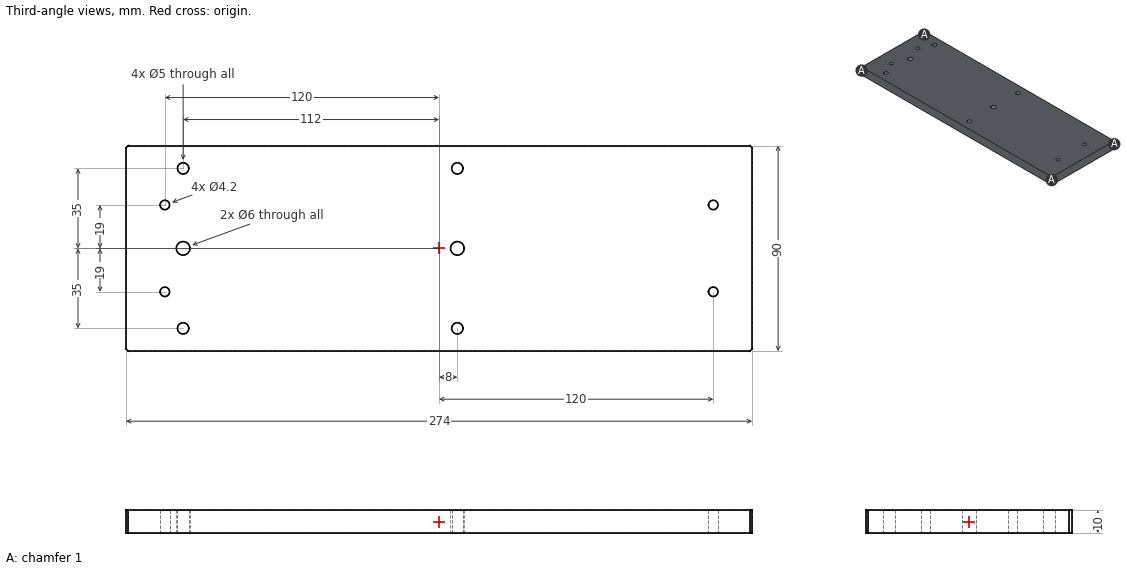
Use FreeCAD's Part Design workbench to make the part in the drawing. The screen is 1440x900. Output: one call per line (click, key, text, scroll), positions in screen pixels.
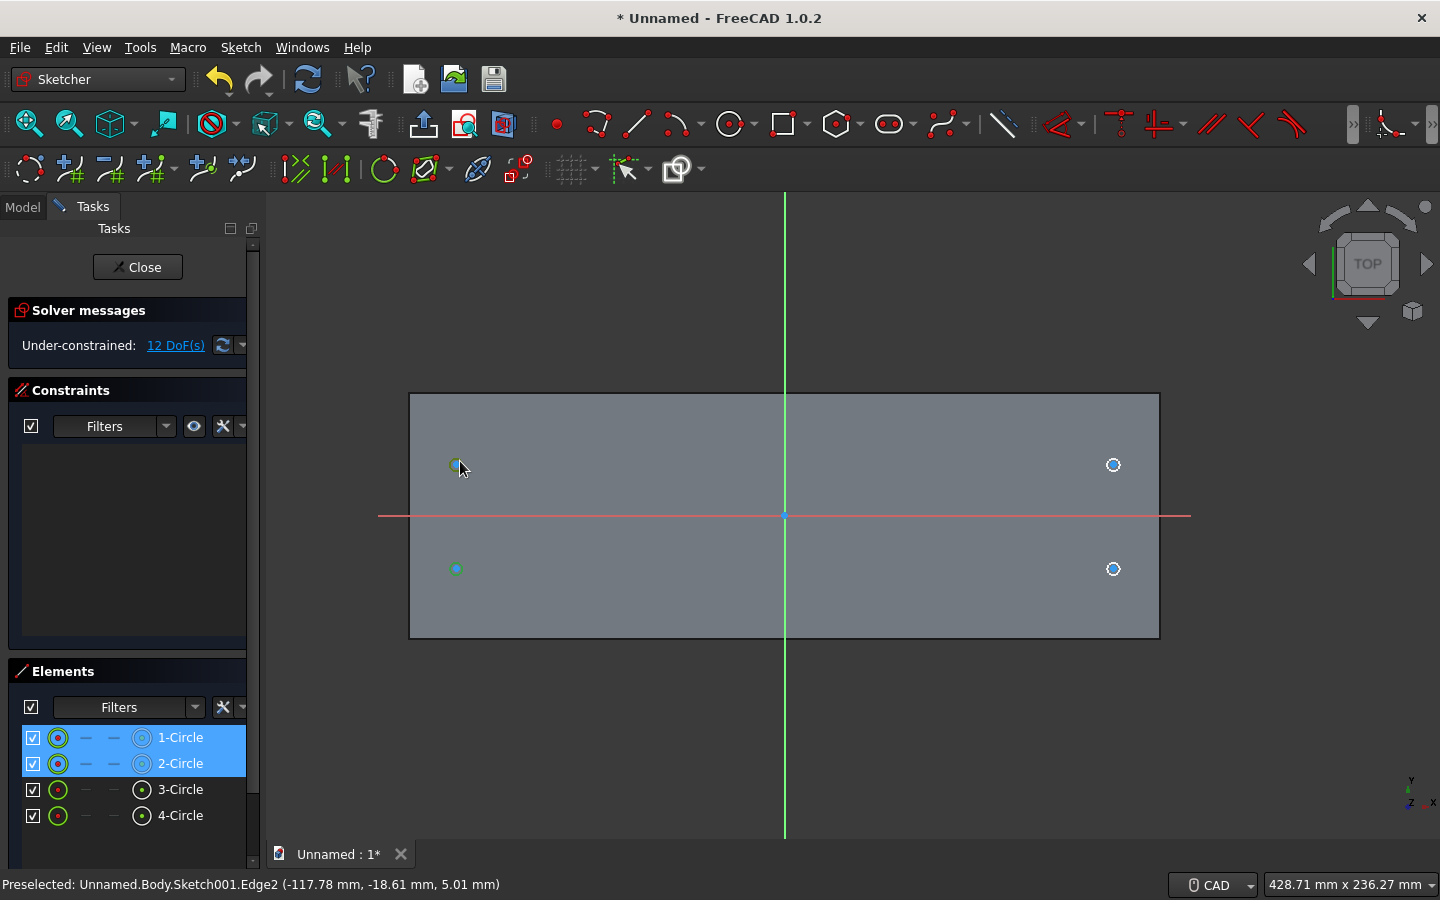
scroll(1118, 565, up, 5)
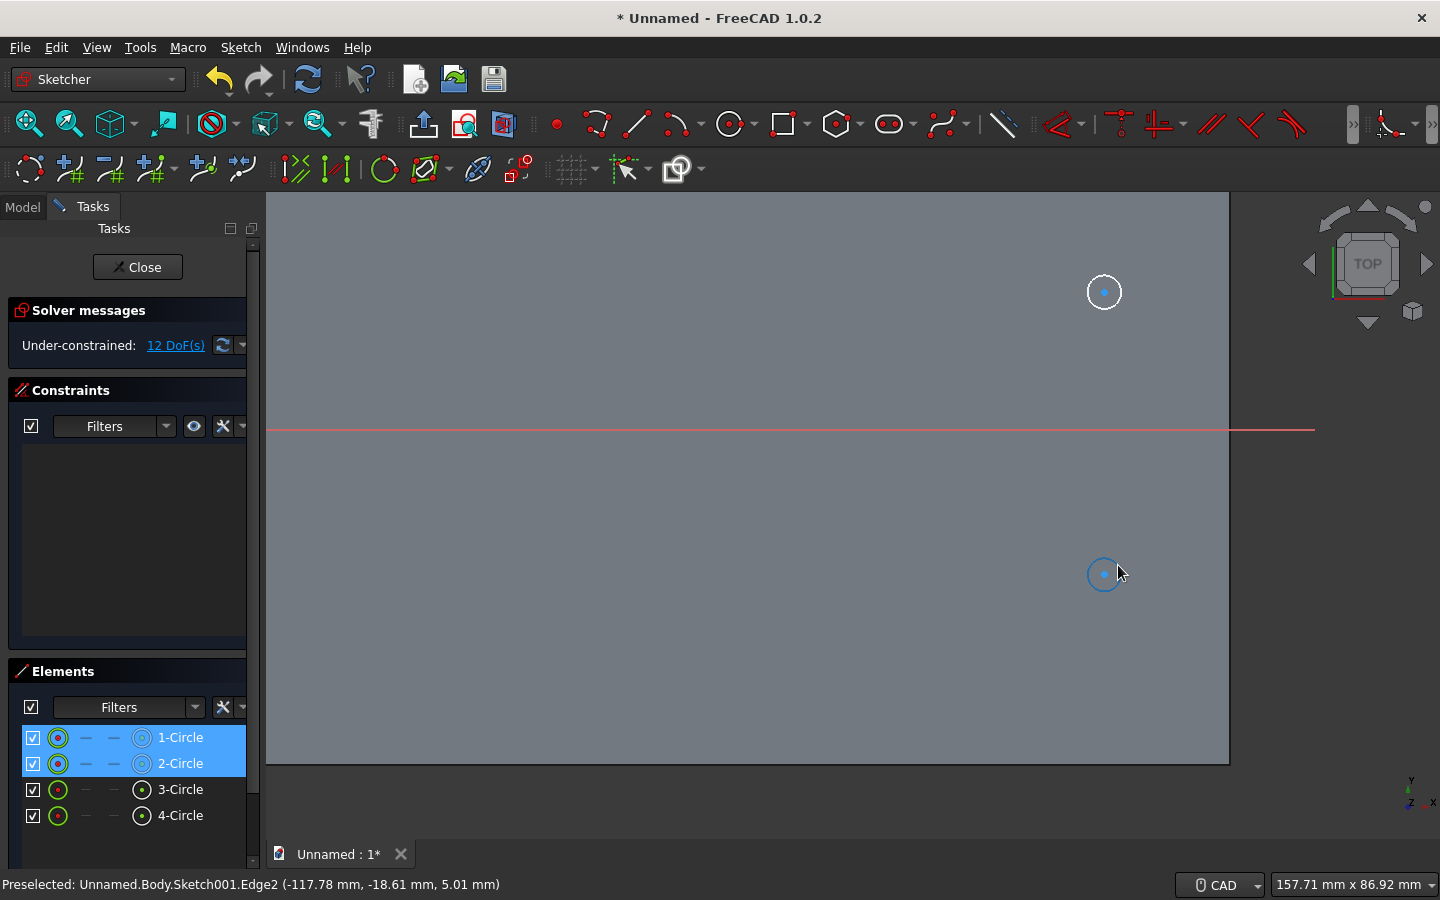
click(1116, 563)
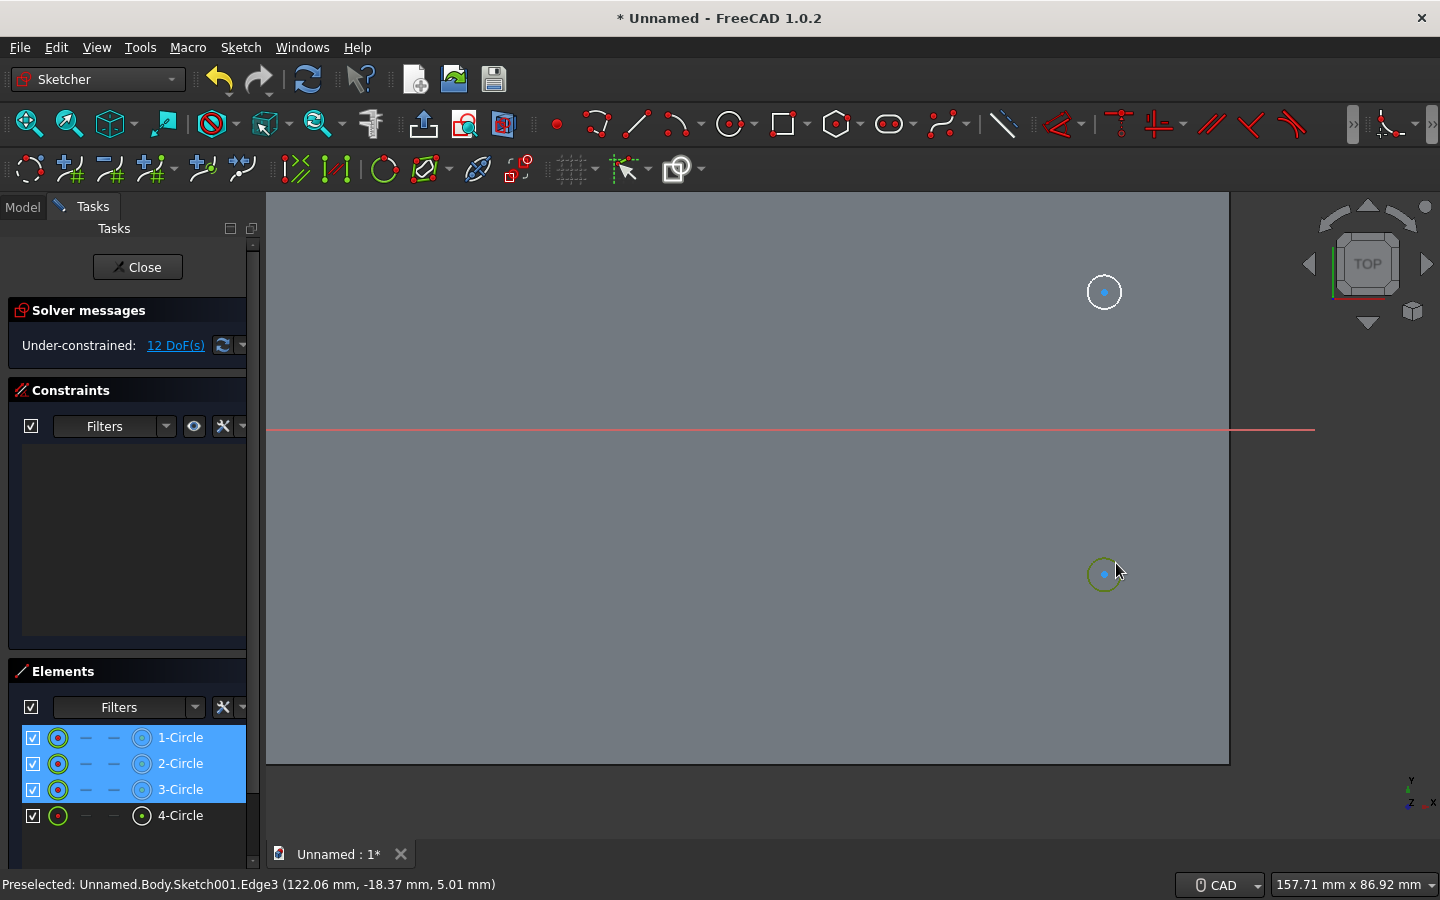
click(1116, 280)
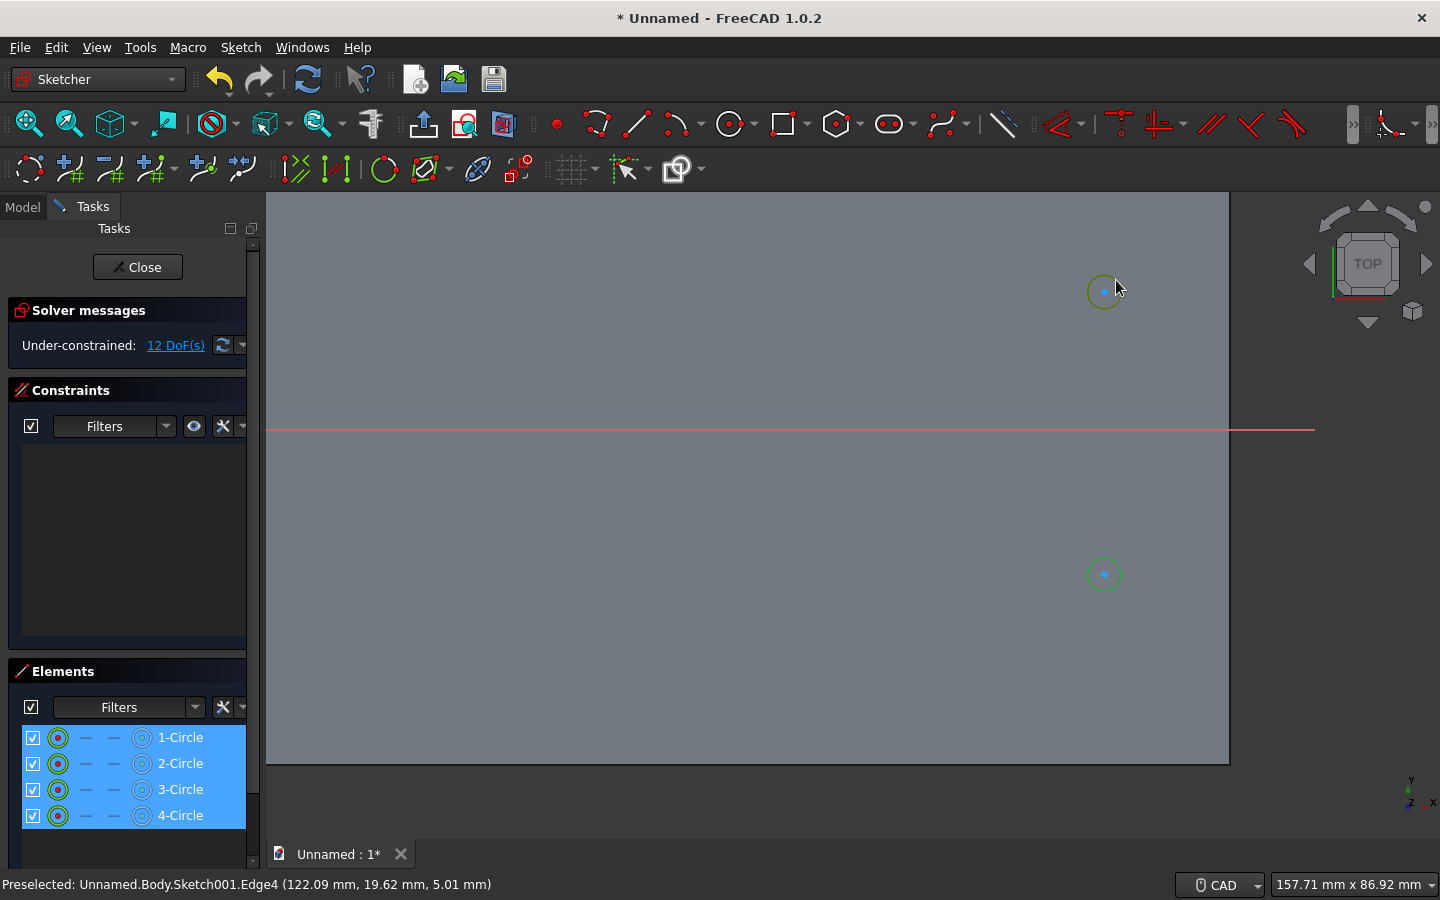
key(e)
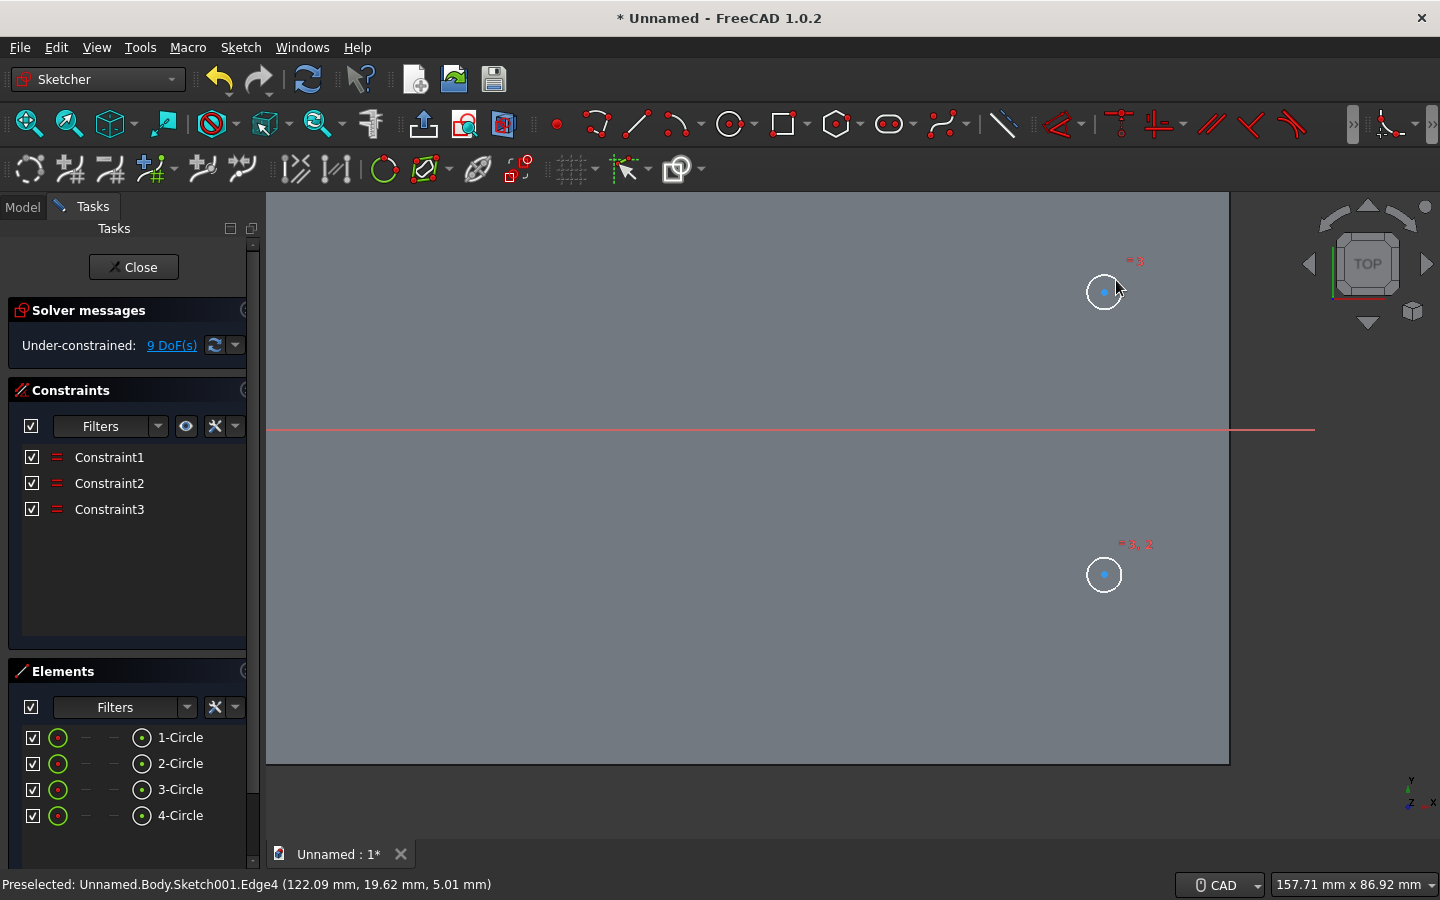
scroll(1119, 565, down, 5)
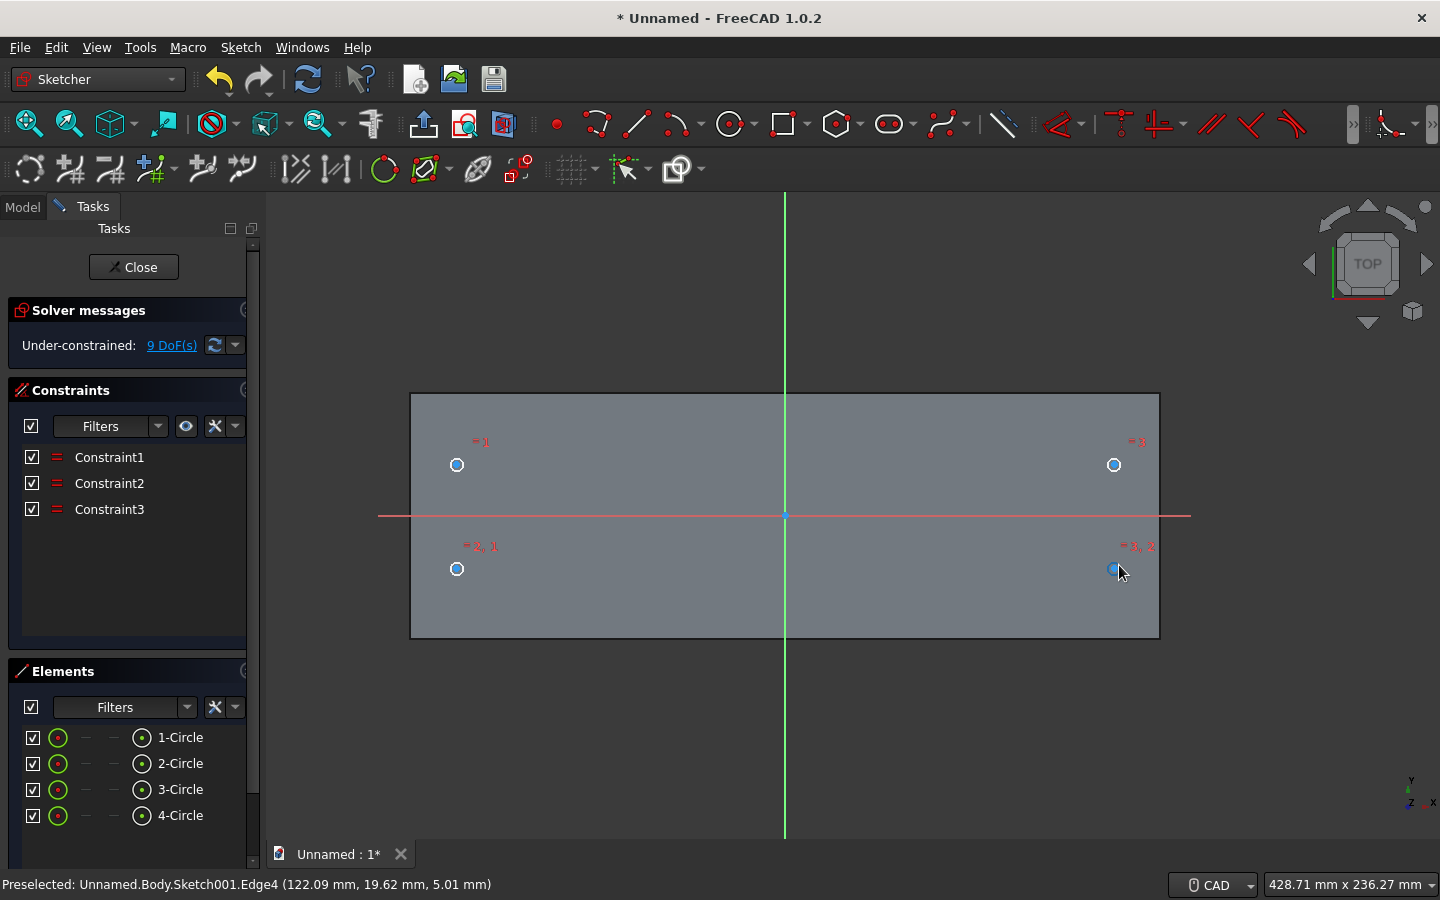
scroll(461, 461, up, 7)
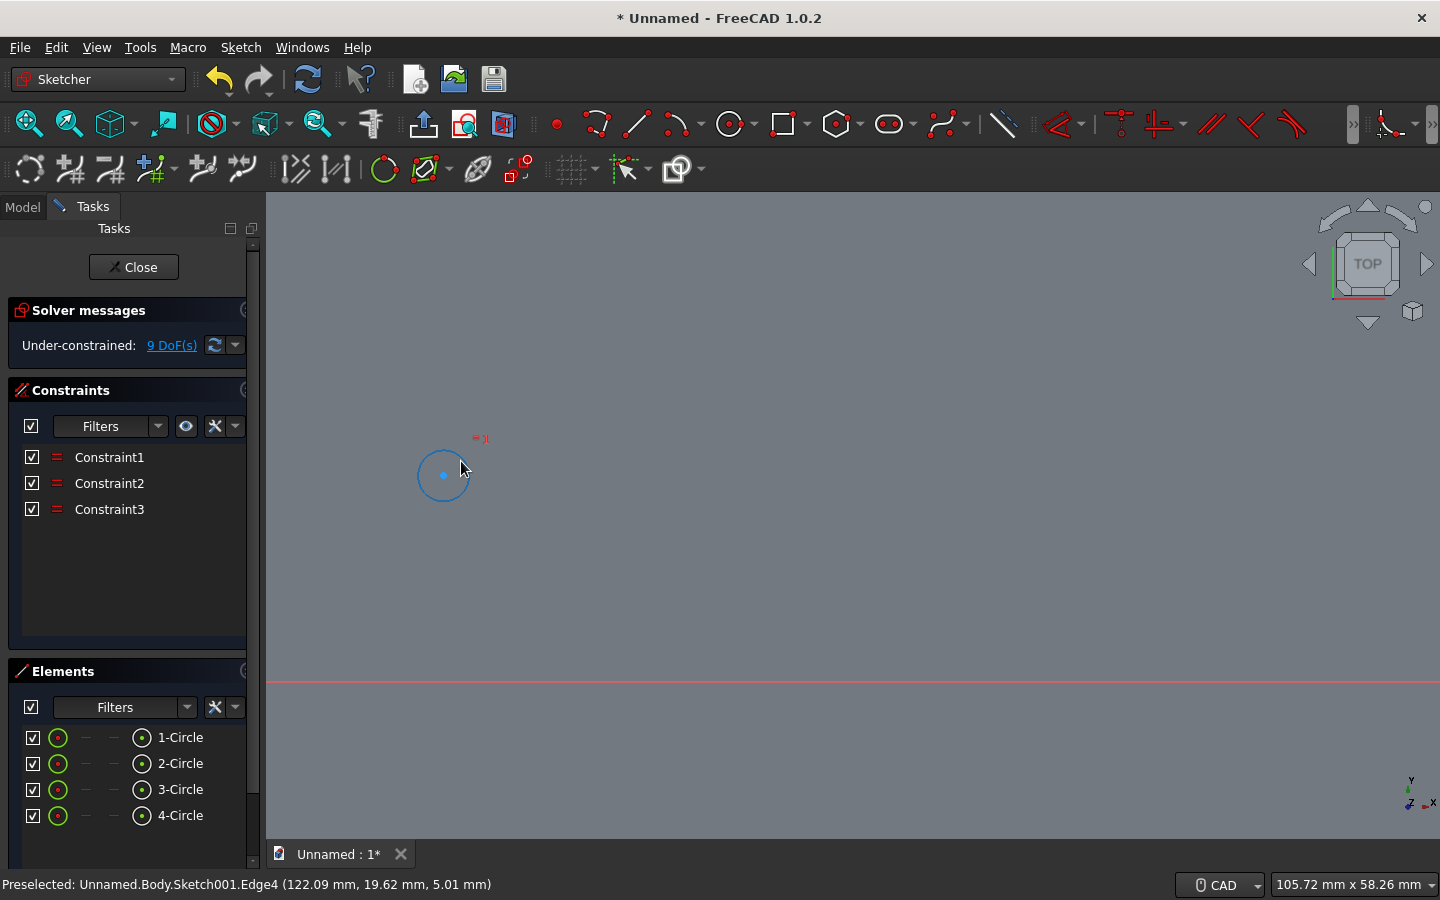
click(462, 458)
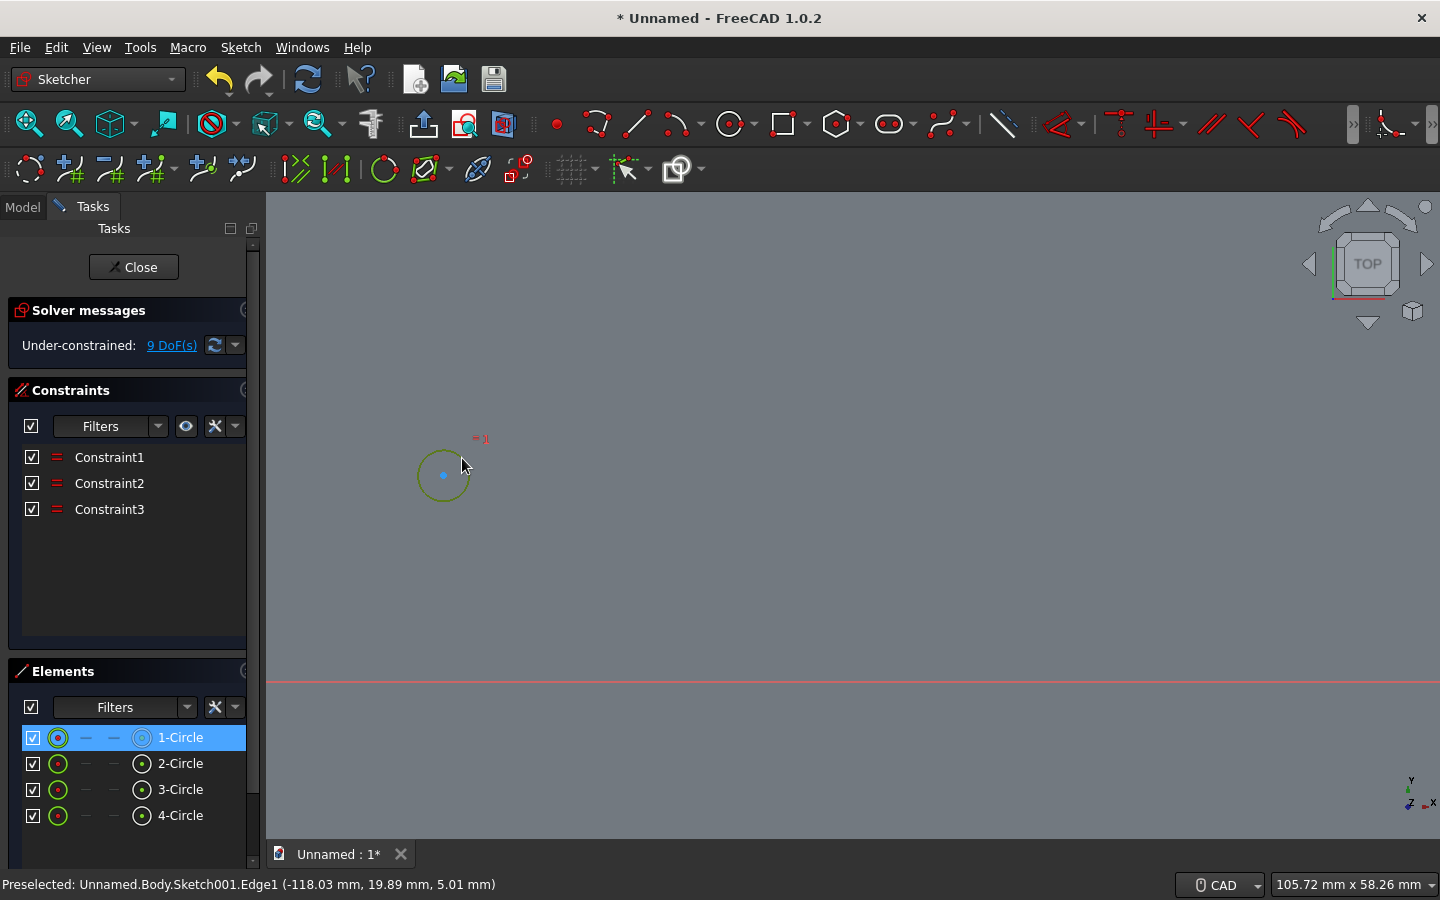
key(k)
key(o)